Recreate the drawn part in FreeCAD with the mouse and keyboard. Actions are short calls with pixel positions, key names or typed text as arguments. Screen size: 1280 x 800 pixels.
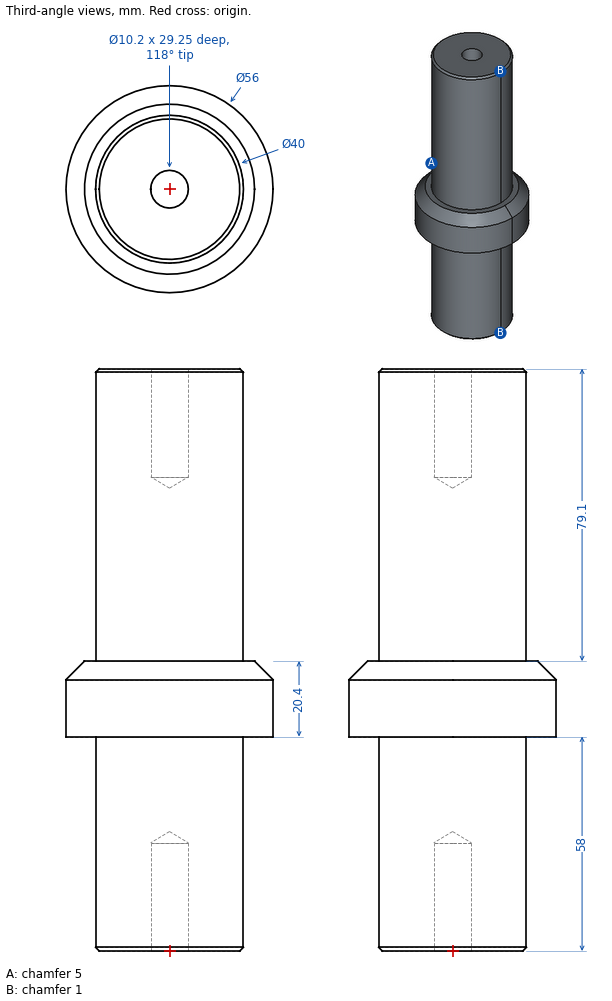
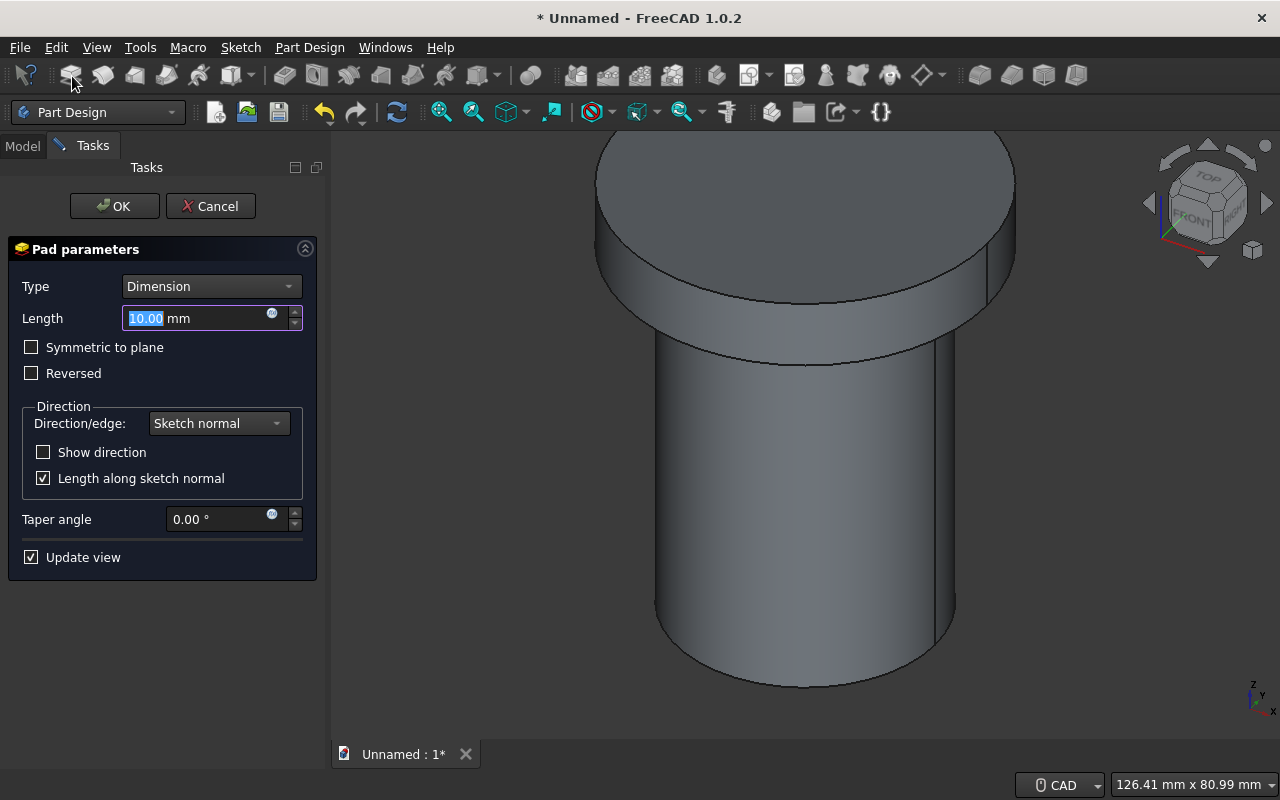
text(20.4)
key(Tab)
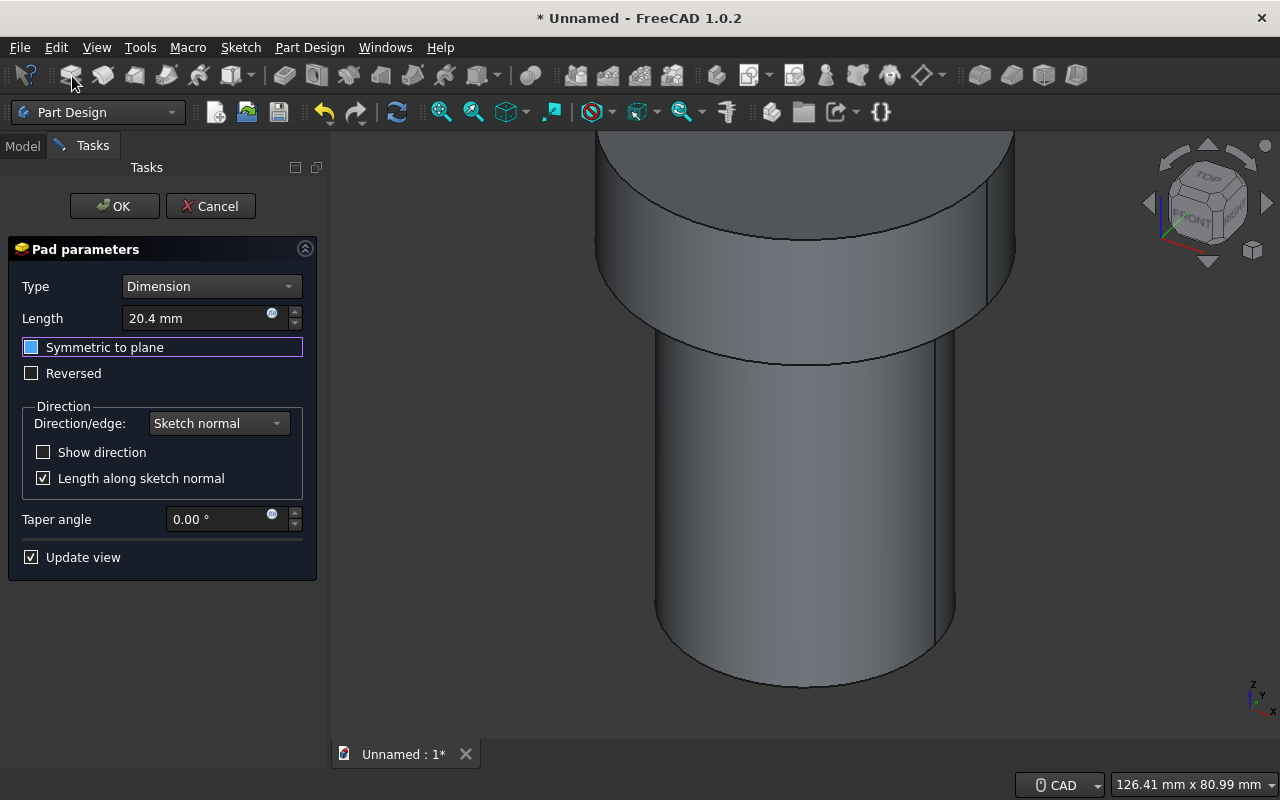
click(115, 206)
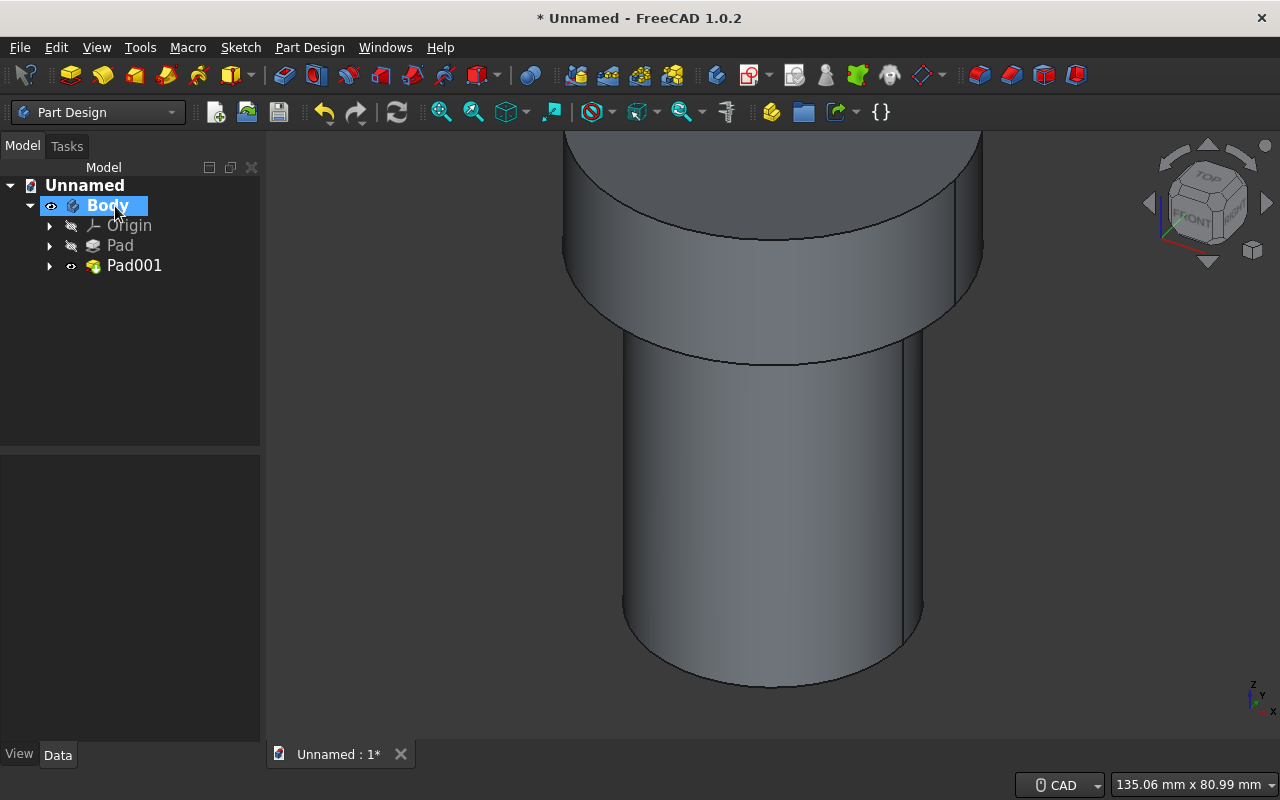
click(442, 112)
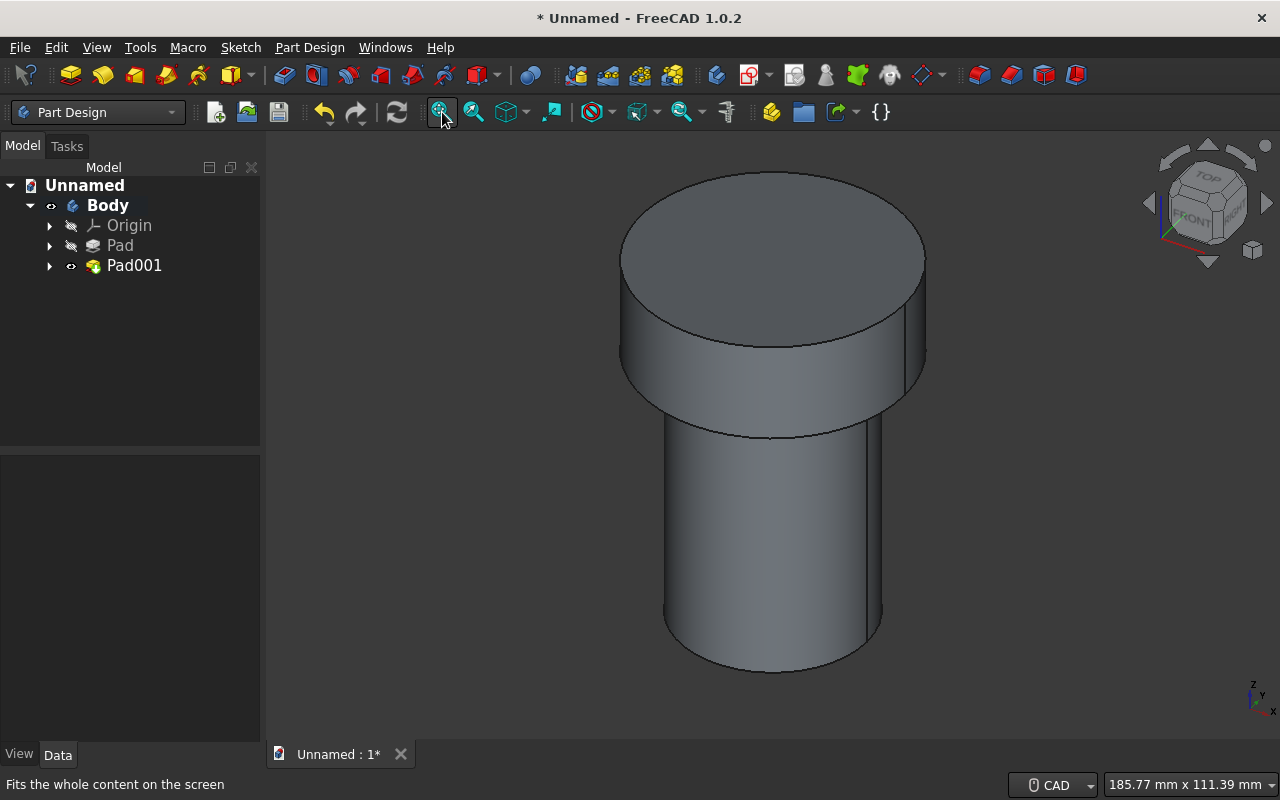
click(773, 259)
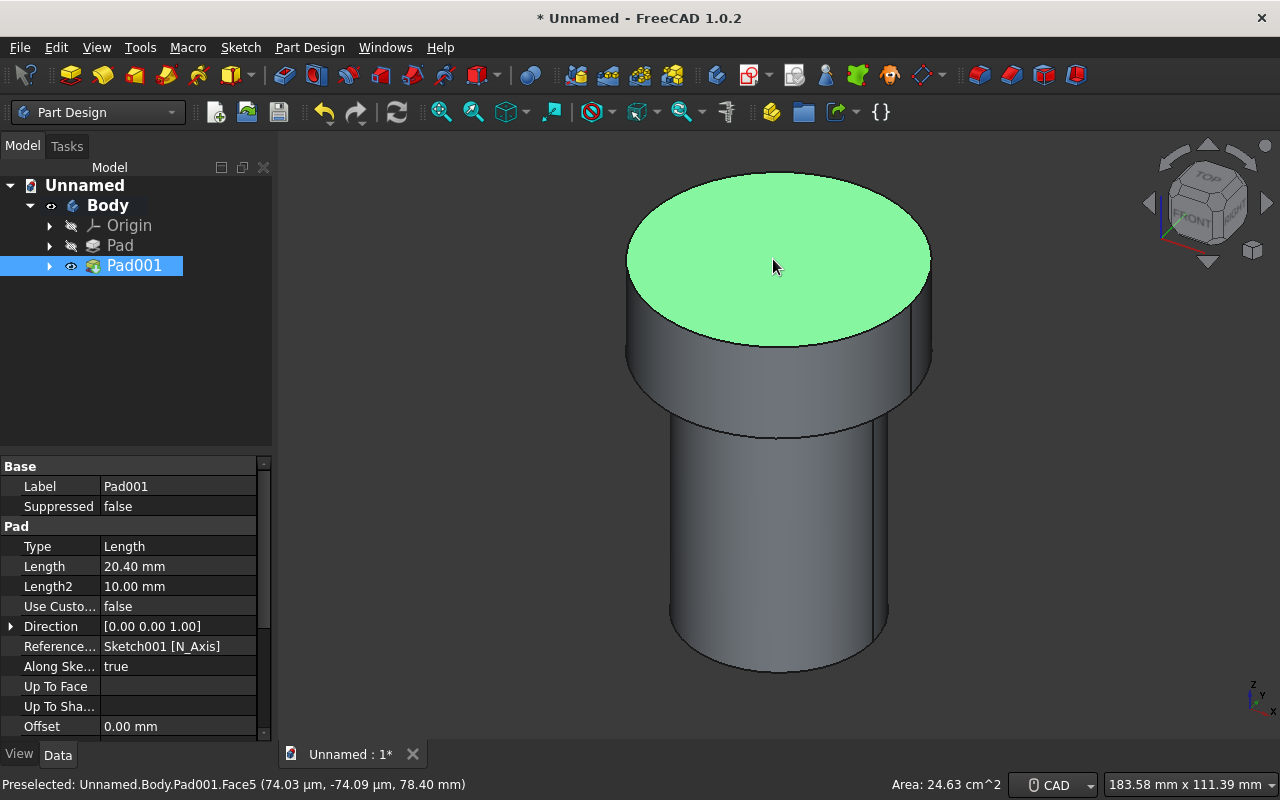
click(750, 76)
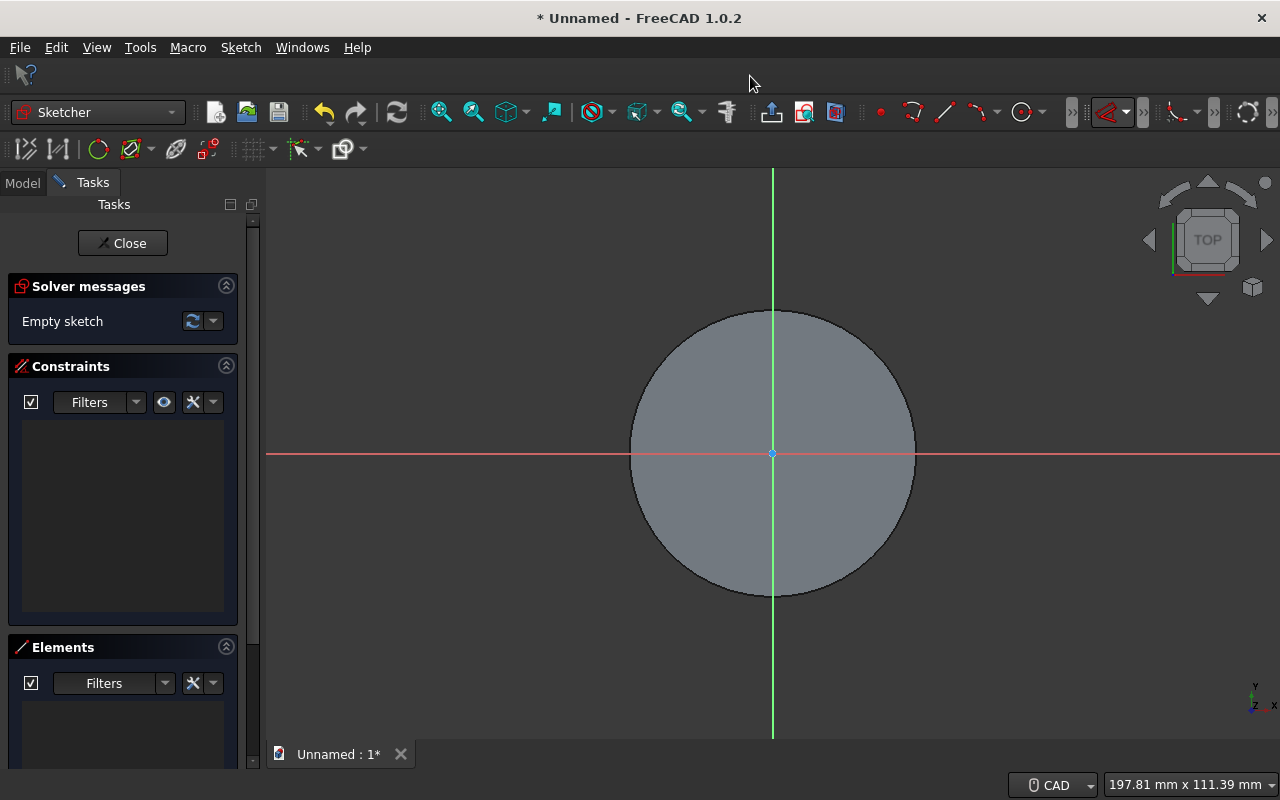
scroll(856, 453, up, 3)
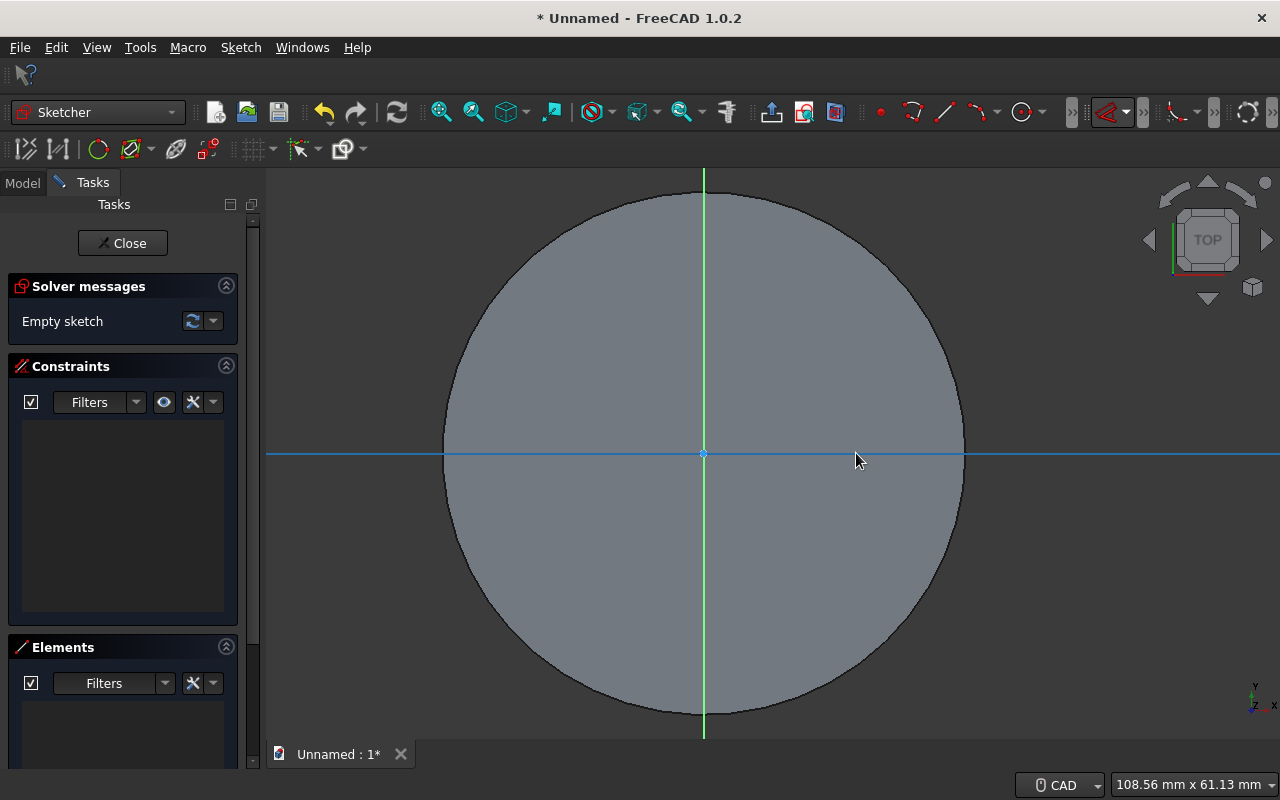
click(1022, 112)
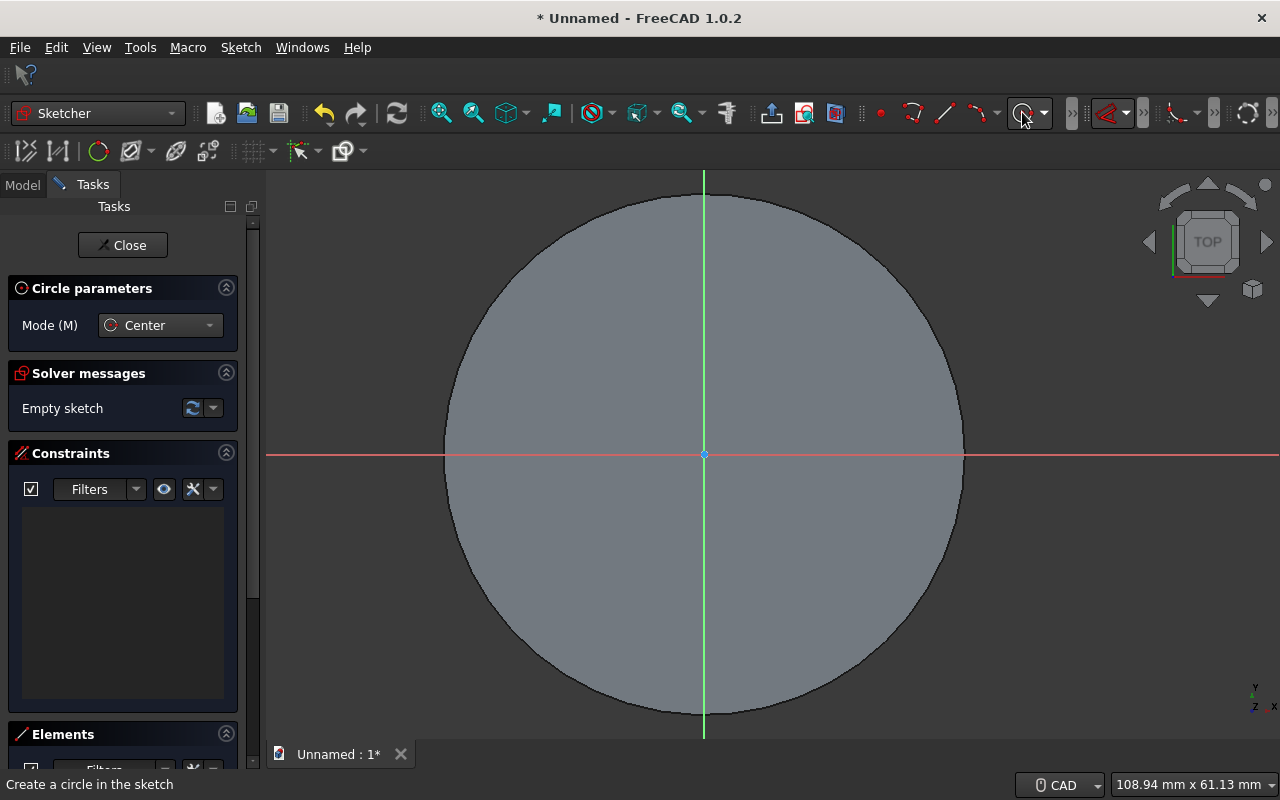
click(704, 454)
move(836, 323)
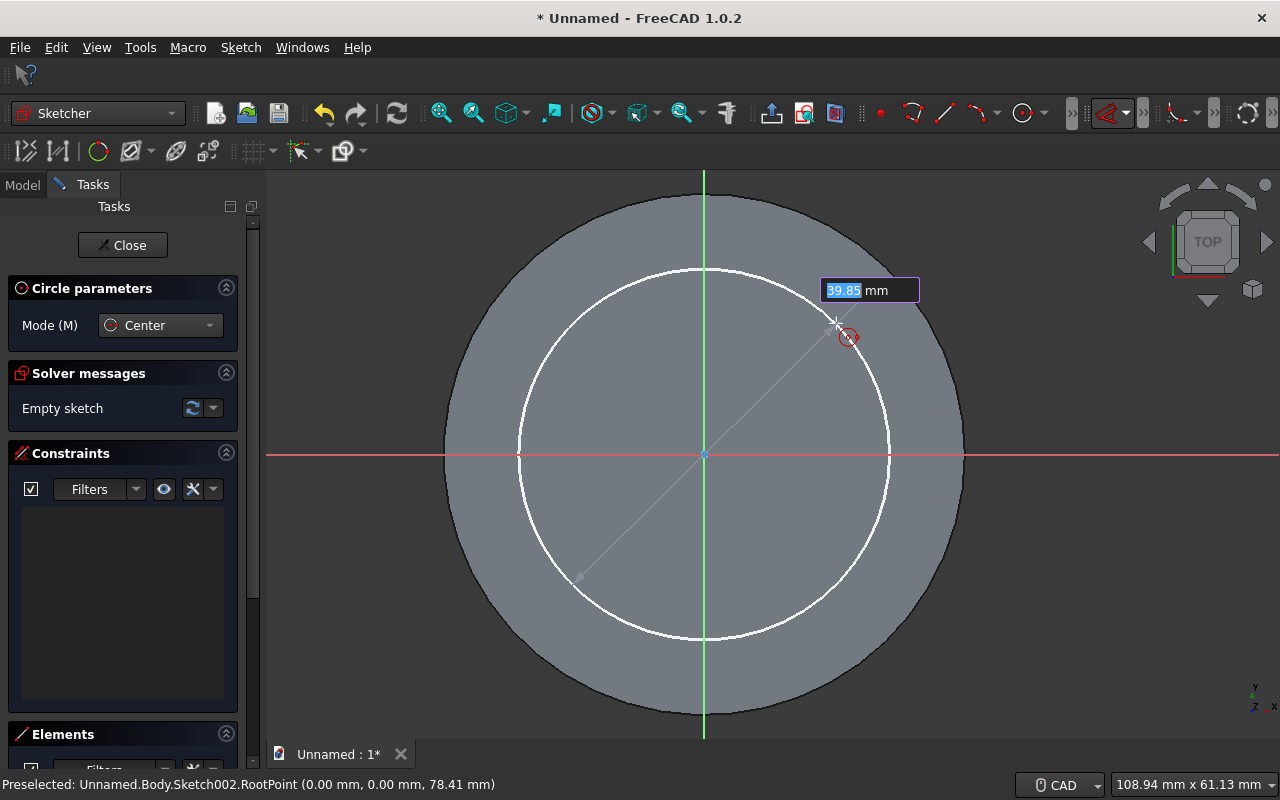
text(40)
key(Return)
key(Escape)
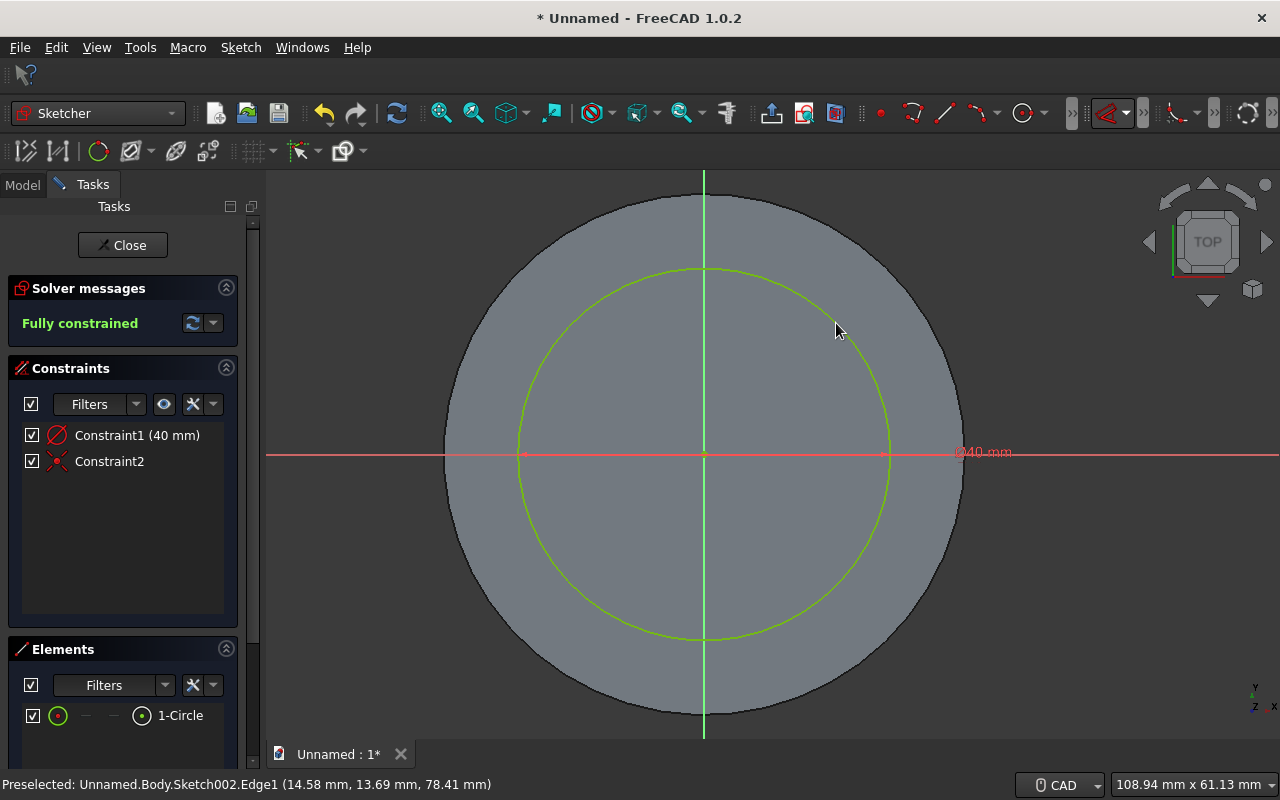
click(123, 245)